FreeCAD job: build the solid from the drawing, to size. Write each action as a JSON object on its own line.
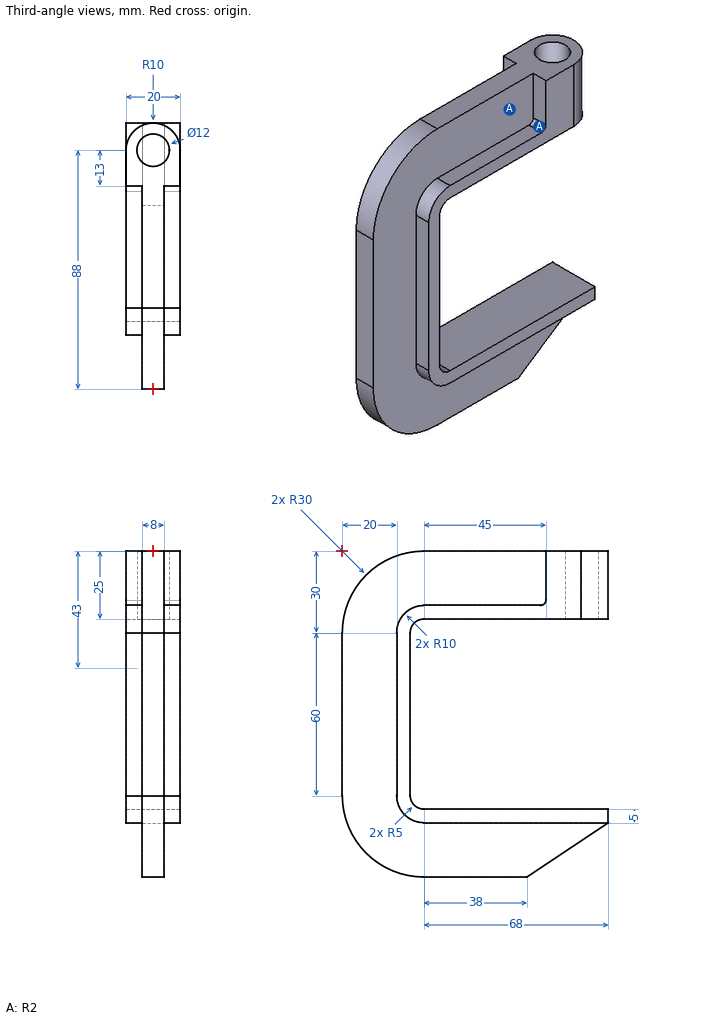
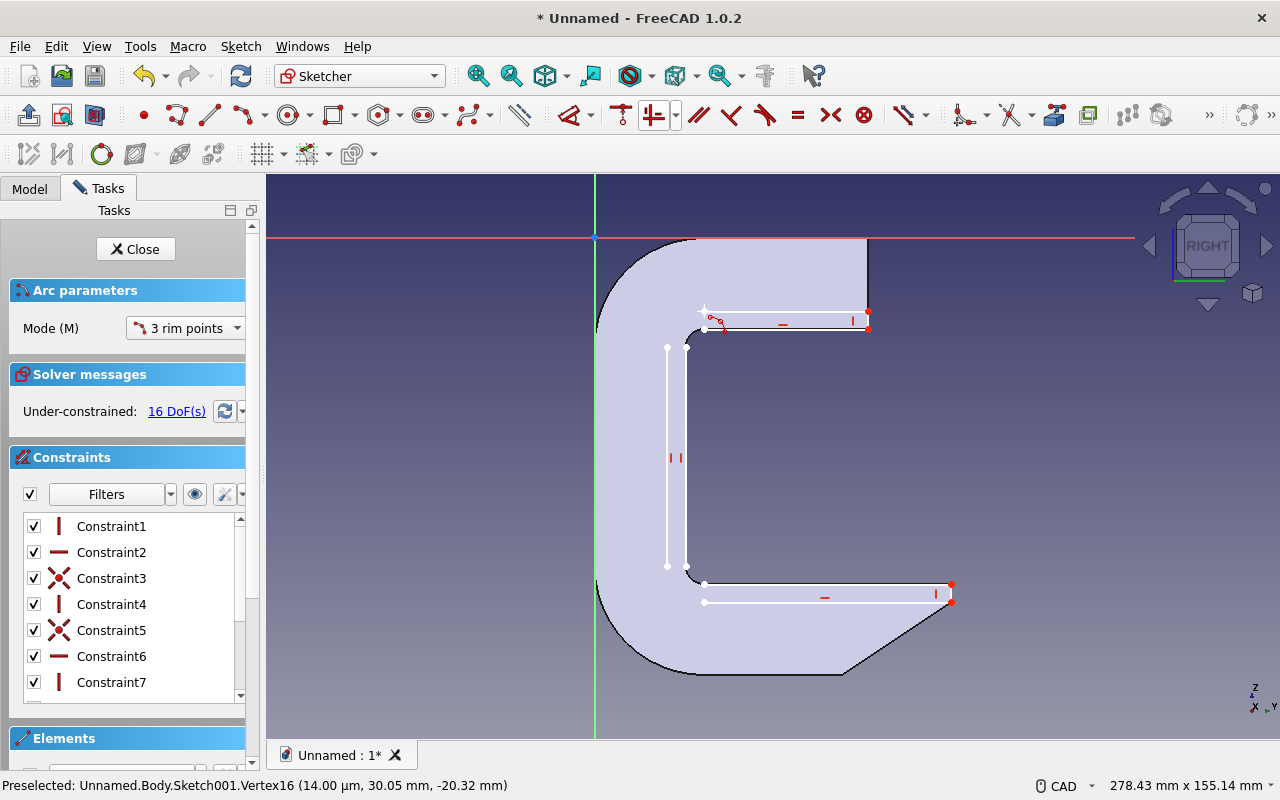
{"action": "left_click", "coordinate": [667, 567]}
{"action": "left_click", "coordinate": [704, 603]}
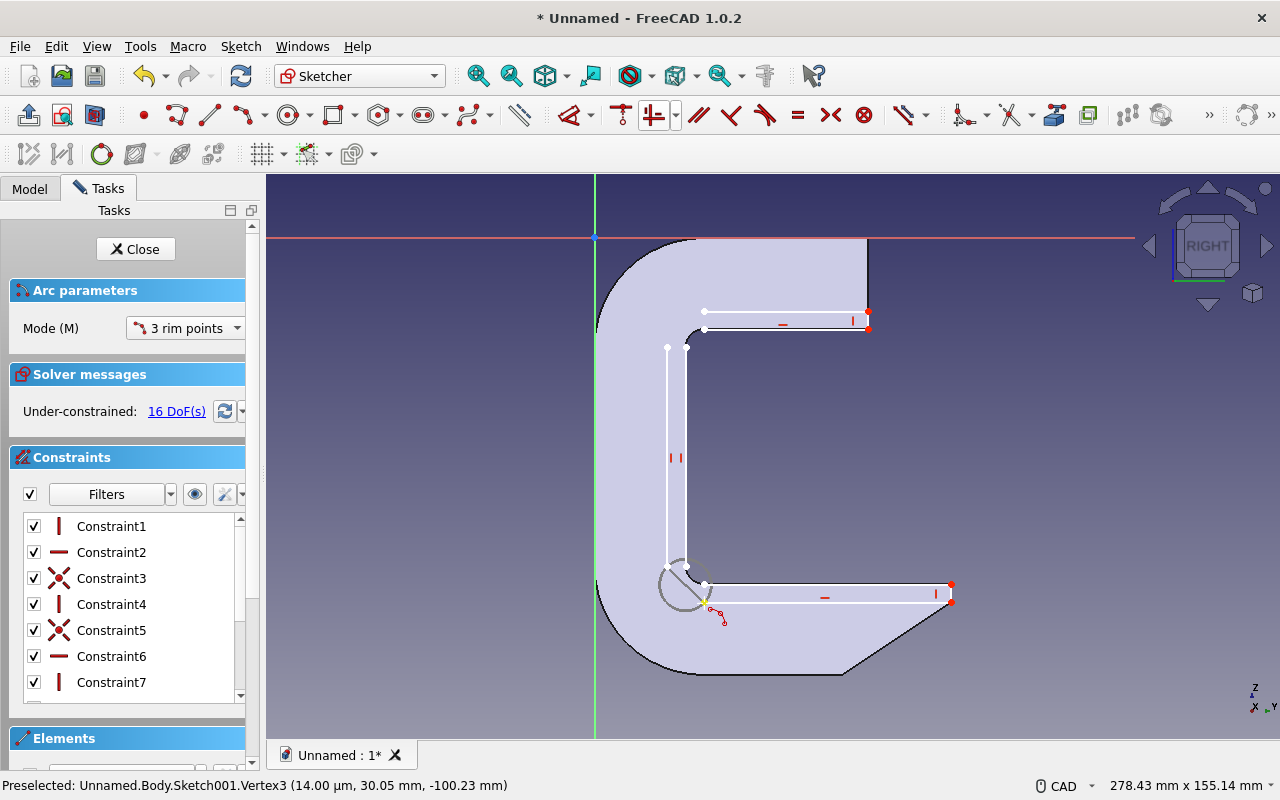
{"action": "scroll", "coordinate": [678, 592], "scroll_direction": "up", "scroll_amount": 2}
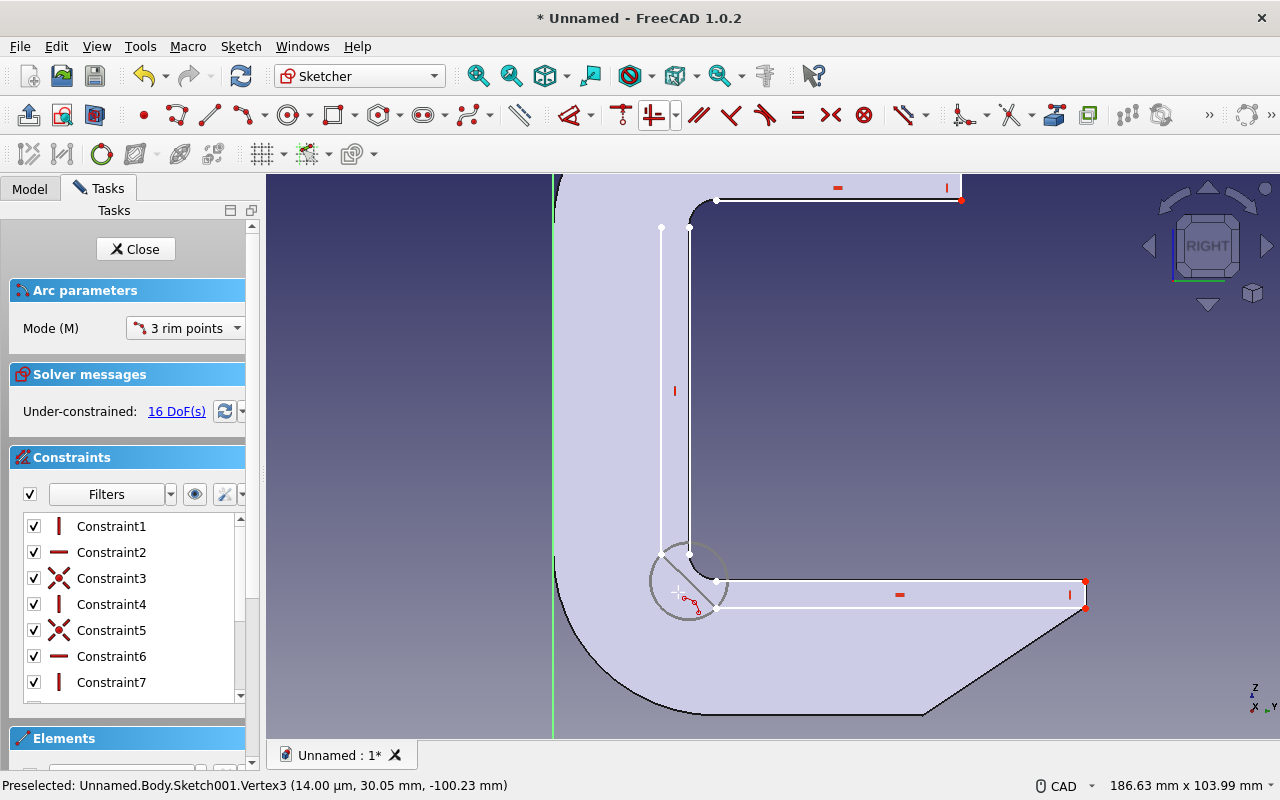
{"action": "left_click", "coordinate": [678, 591]}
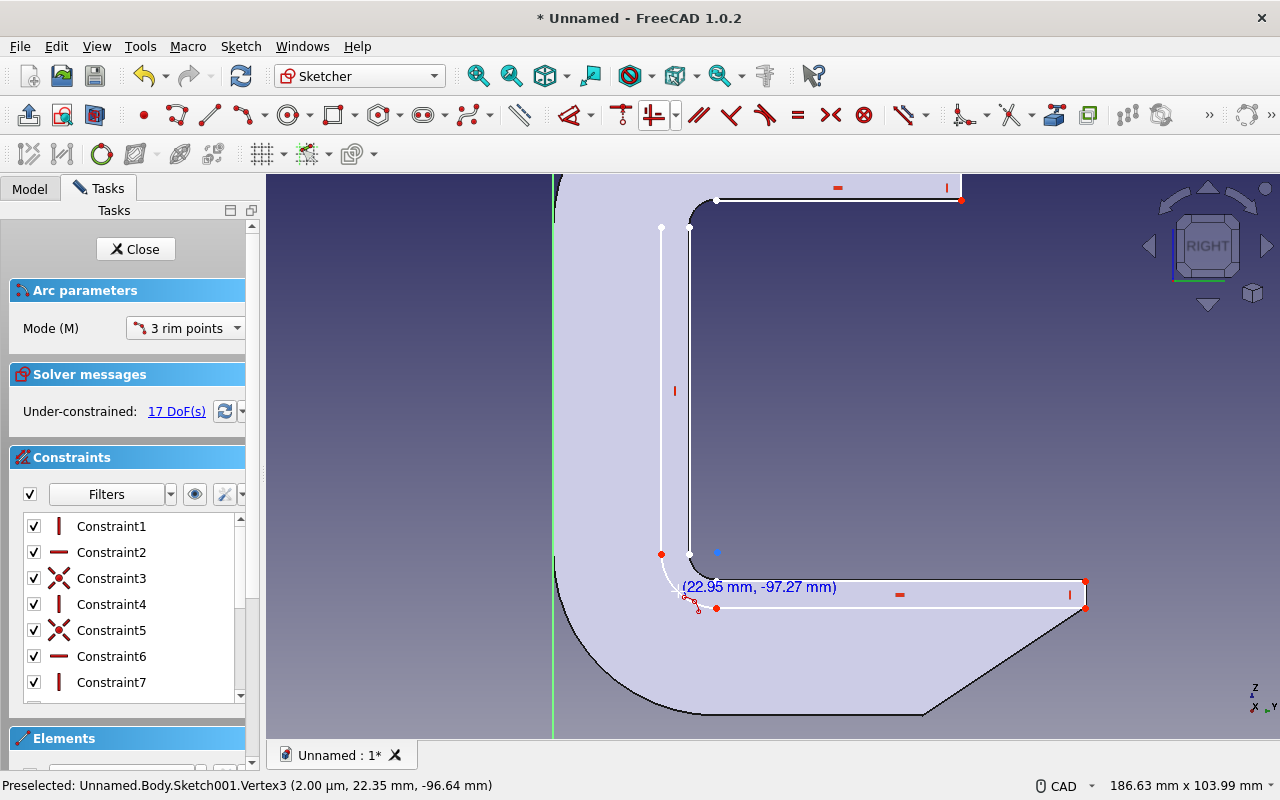
{"action": "left_click", "coordinate": [717, 581]}
{"action": "left_click", "coordinate": [690, 554]}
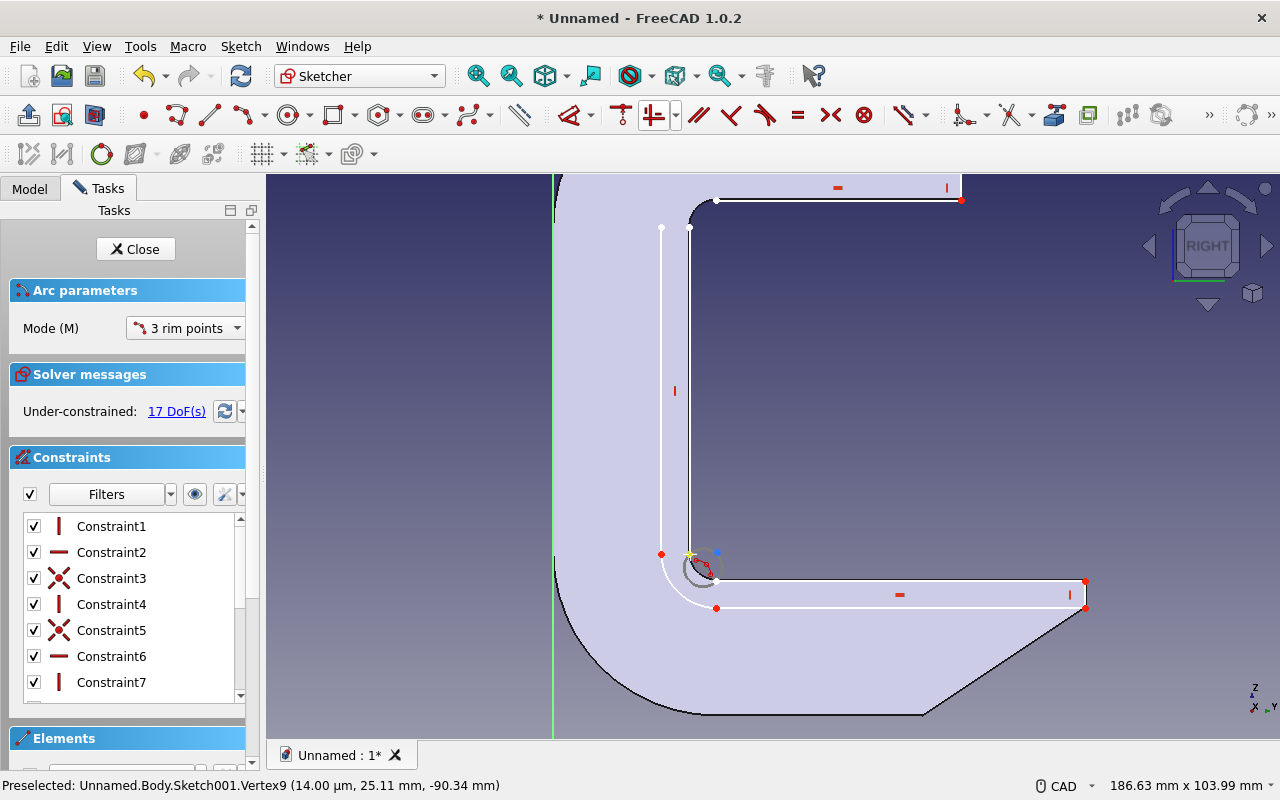
{"action": "scroll", "coordinate": [697, 572], "scroll_direction": "up", "scroll_amount": 4}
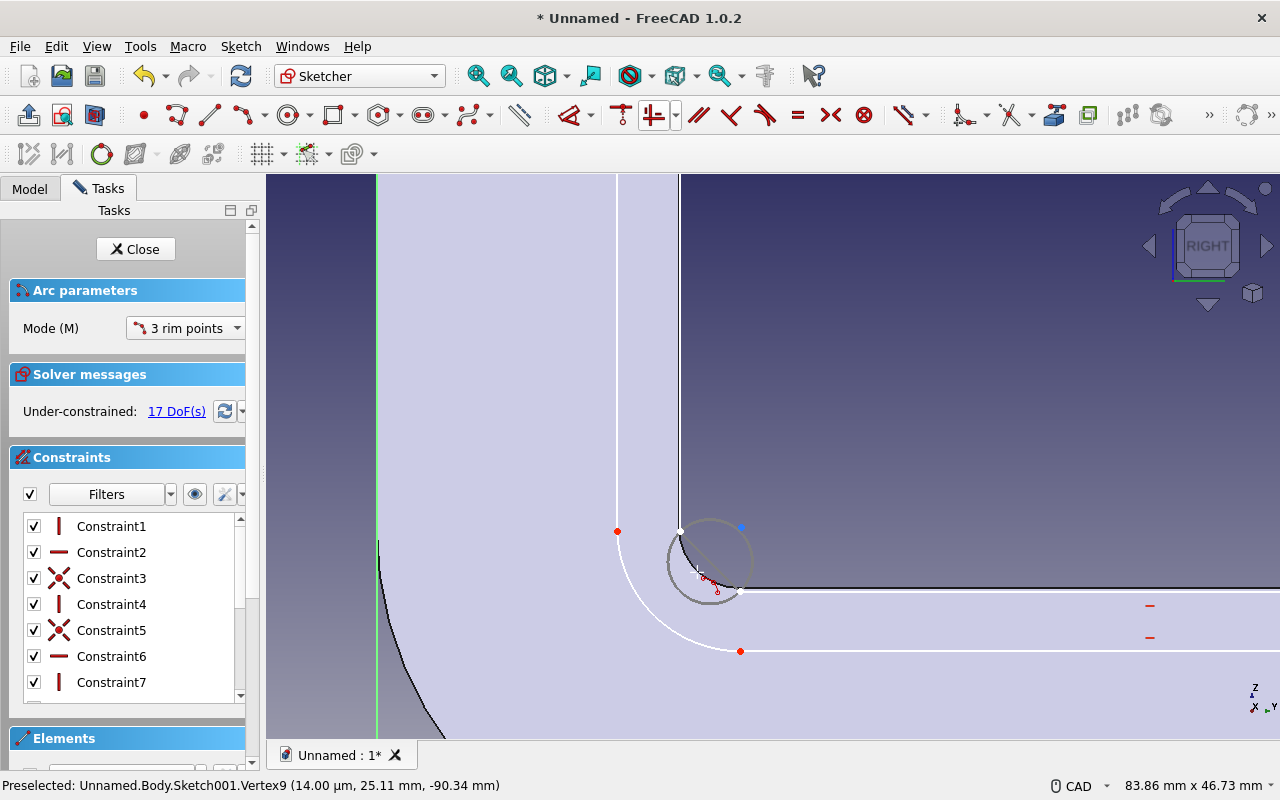
{"action": "left_click", "coordinate": [697, 570]}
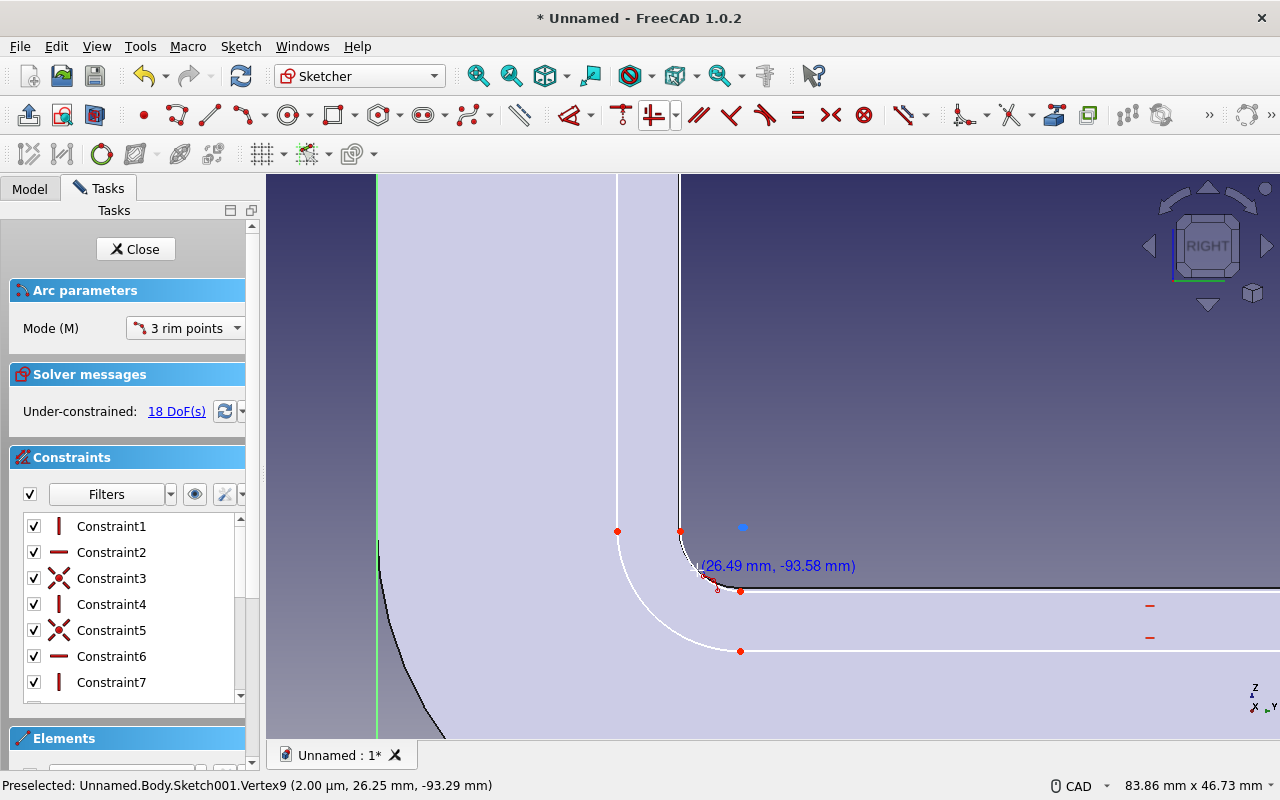
{"action": "scroll", "coordinate": [590, 634], "scroll_direction": "down", "scroll_amount": 6}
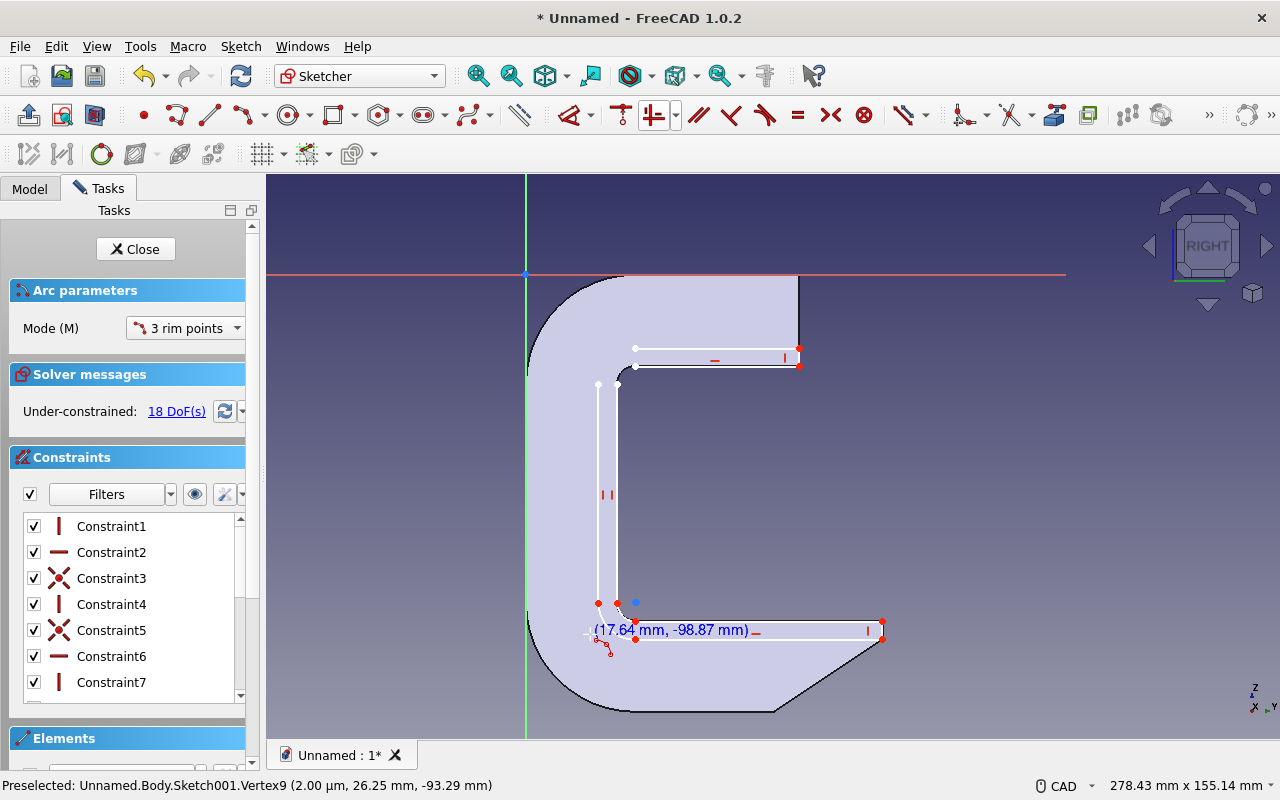
{"action": "left_click", "coordinate": [617, 385]}
{"action": "left_click", "coordinate": [635, 367]}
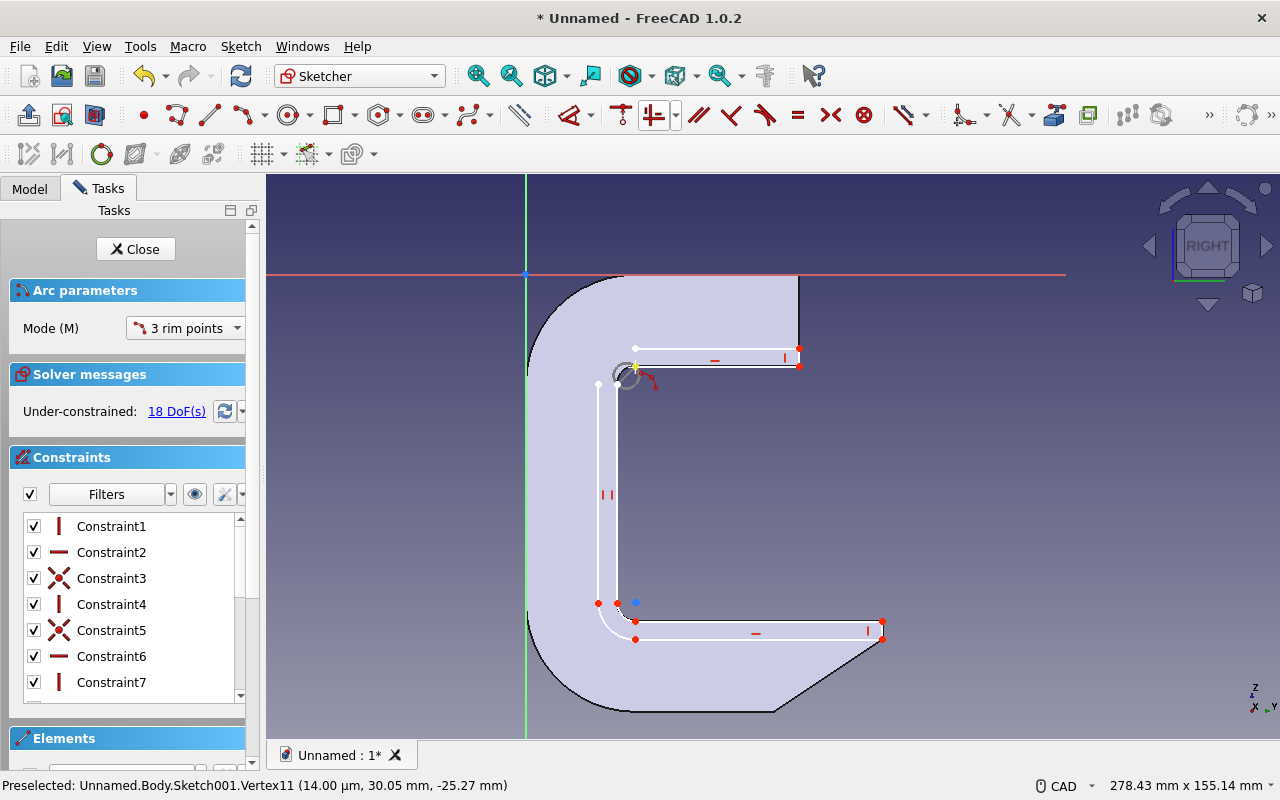
{"action": "scroll", "coordinate": [622, 371], "scroll_direction": "up", "scroll_amount": 6}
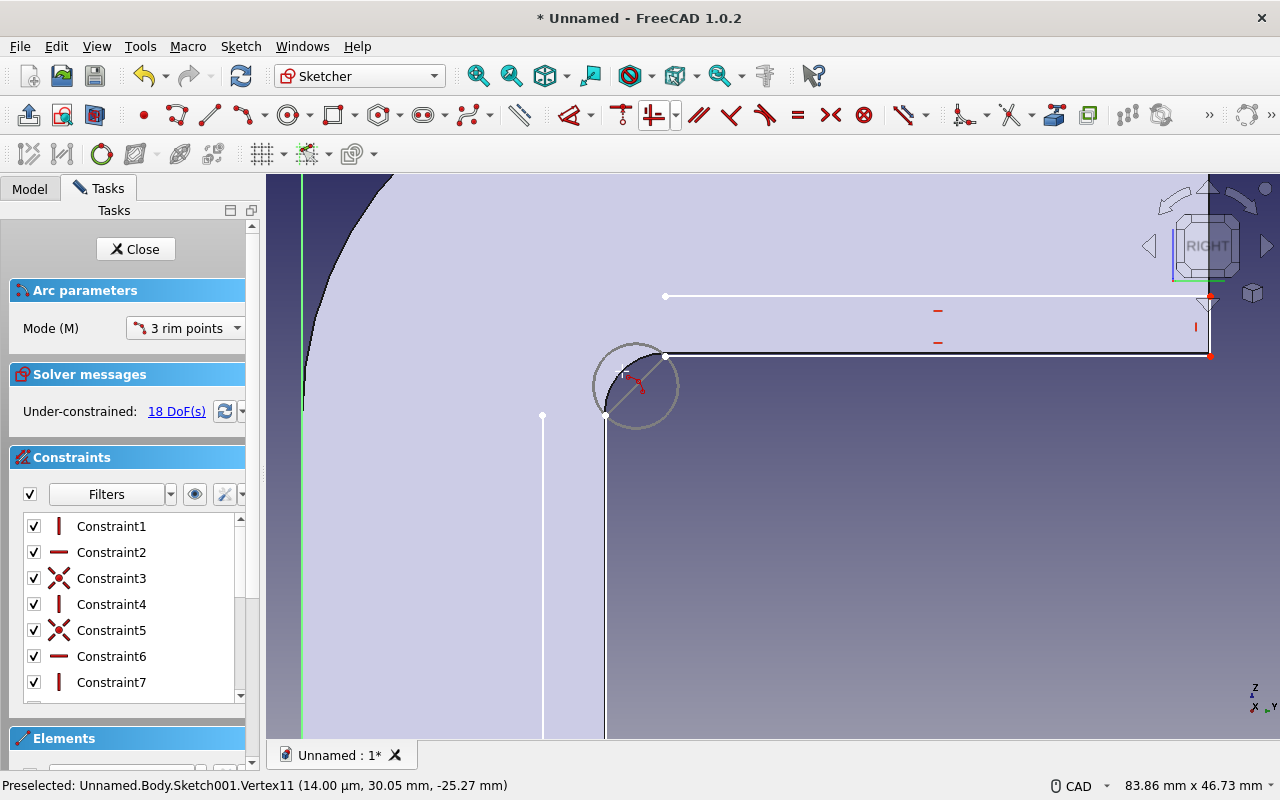
{"action": "left_click", "coordinate": [622, 371]}